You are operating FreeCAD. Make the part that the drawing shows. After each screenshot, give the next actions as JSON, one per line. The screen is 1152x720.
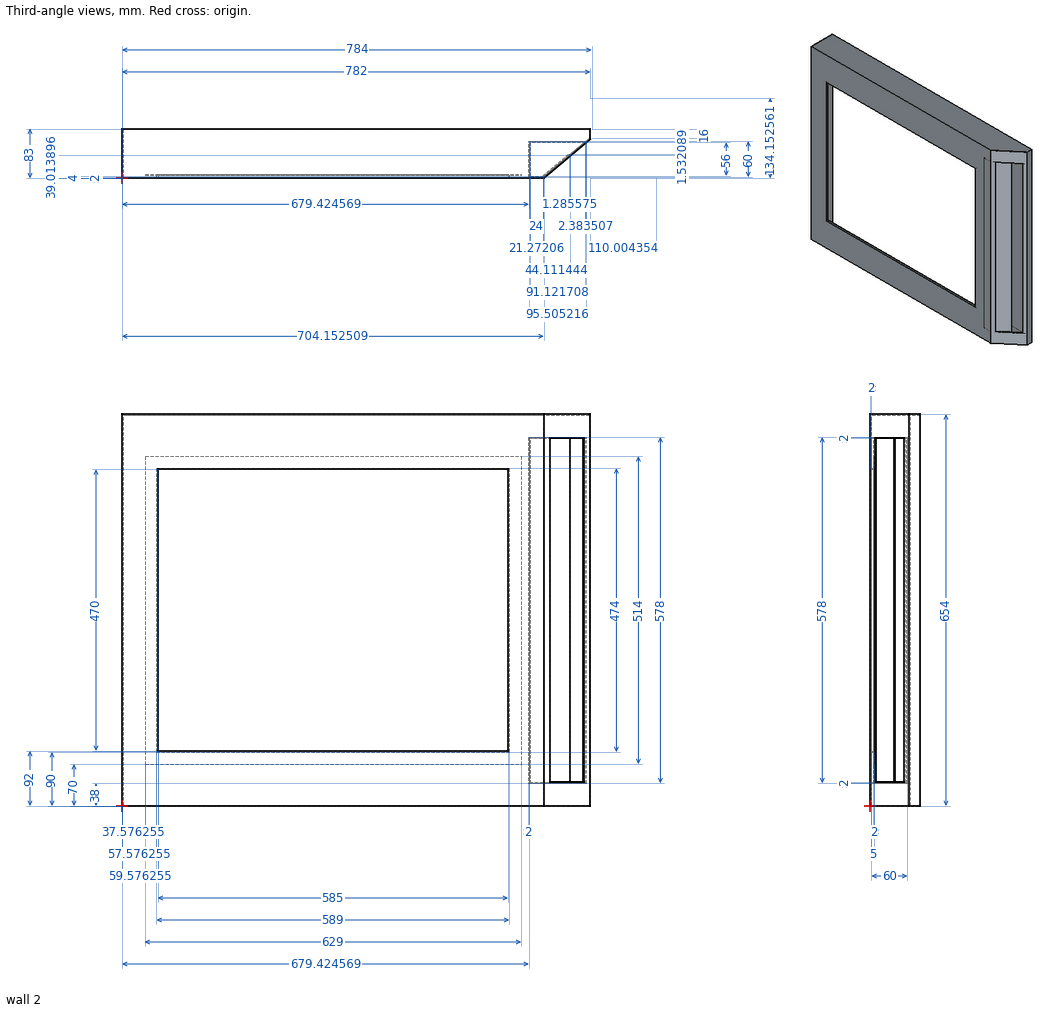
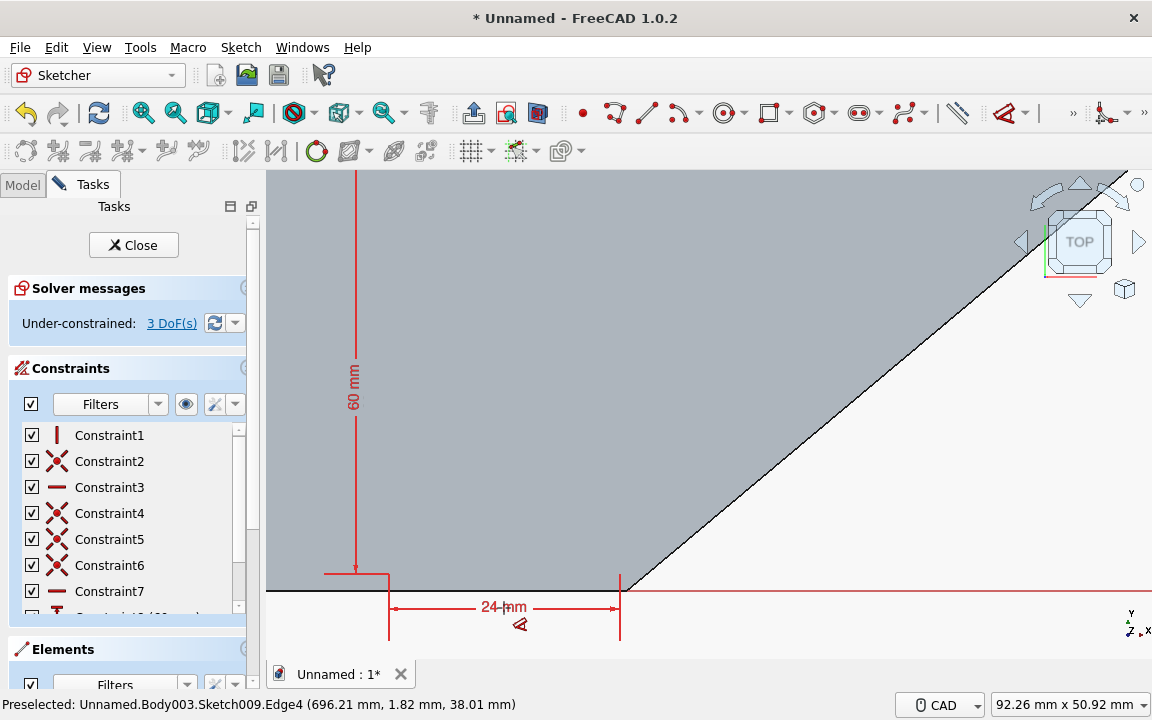
{"action": "scroll", "coordinate": [389, 574], "scroll_direction": "up", "scroll_amount": 4}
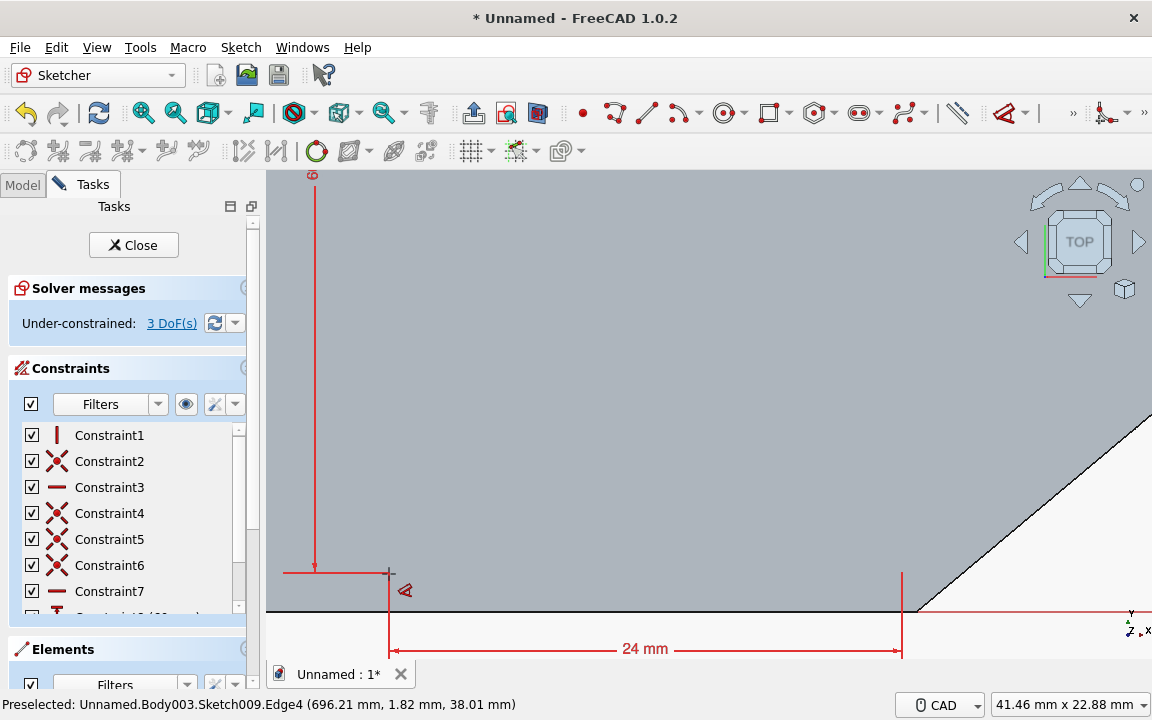
{"action": "left_click", "coordinate": [389, 573]}
{"action": "left_click", "coordinate": [423, 592]}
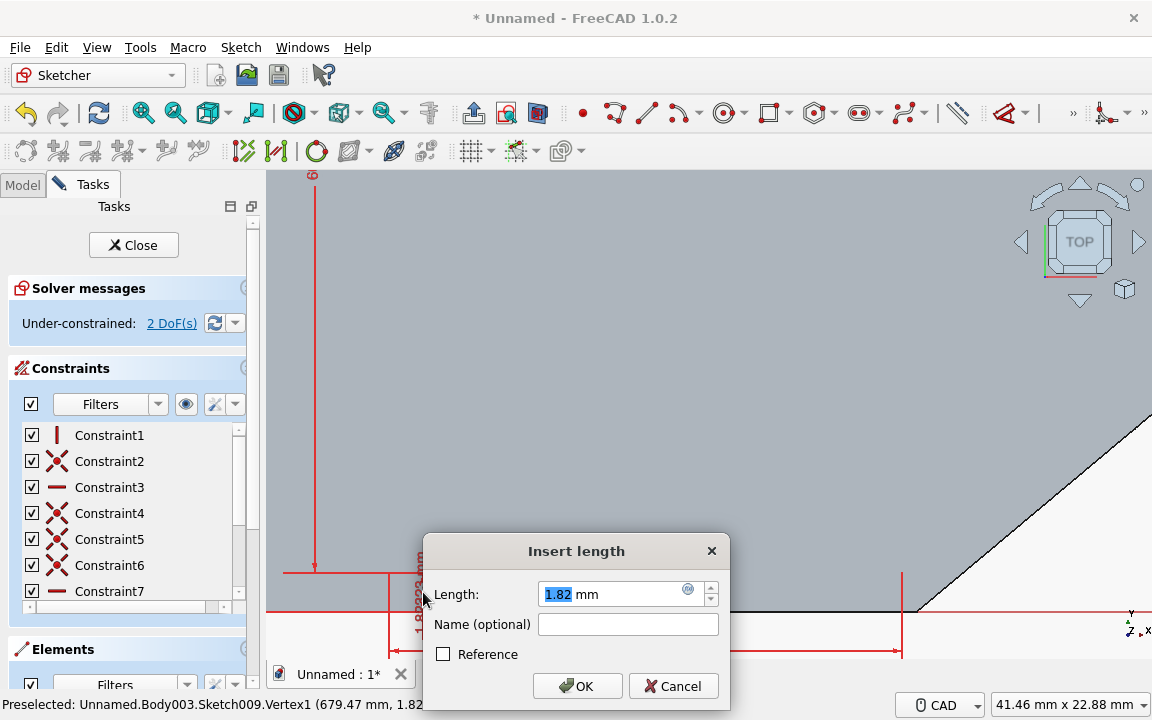
{"action": "type", "text": "2"}
{"action": "key", "text": "Return"}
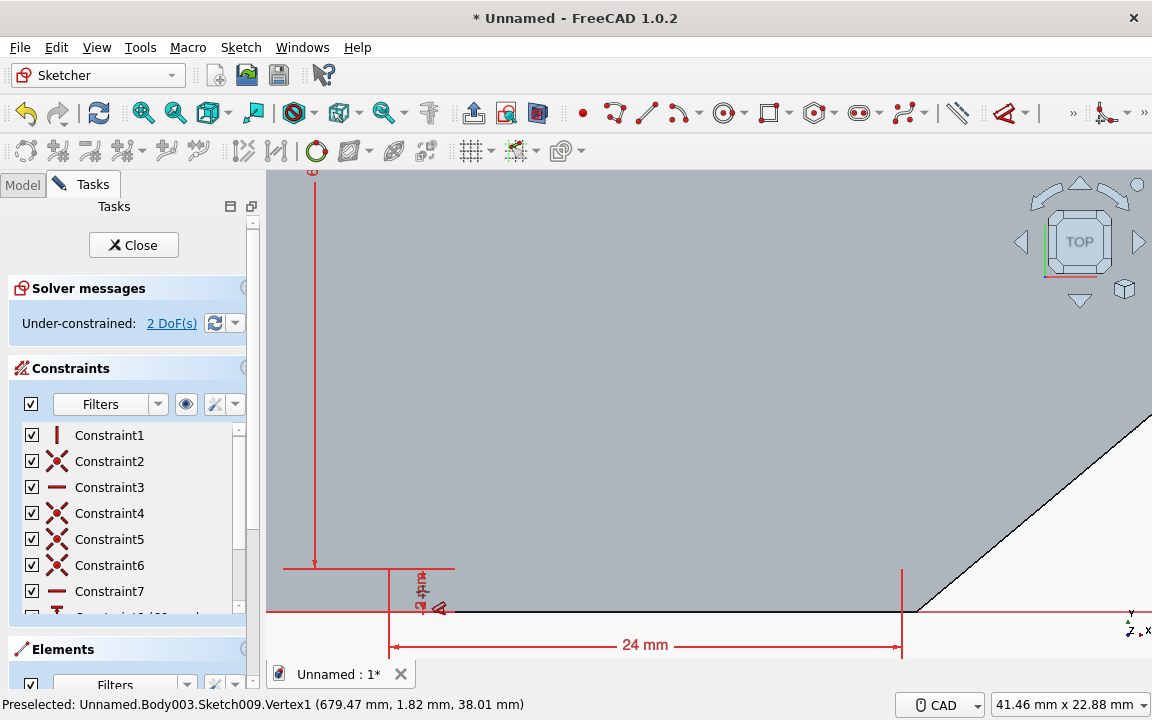
{"action": "scroll", "coordinate": [389, 574], "scroll_direction": "down", "scroll_amount": 7}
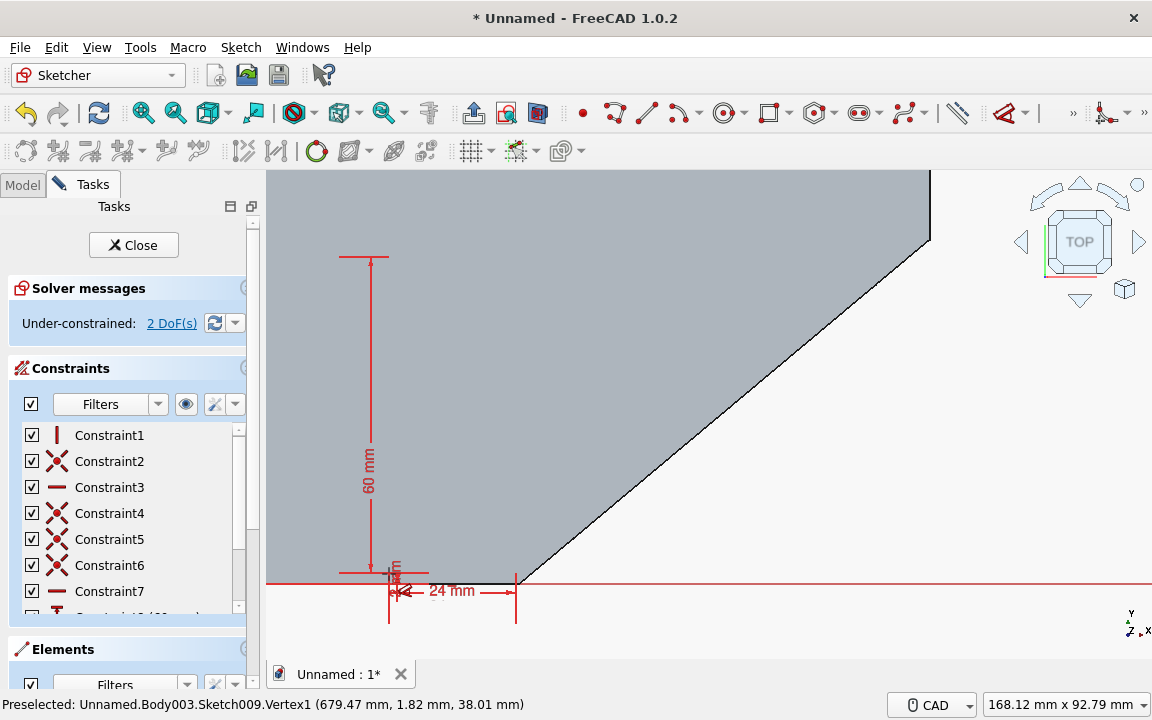
{"action": "left_click", "coordinate": [540, 257]}
{"action": "left_click", "coordinate": [641, 223]}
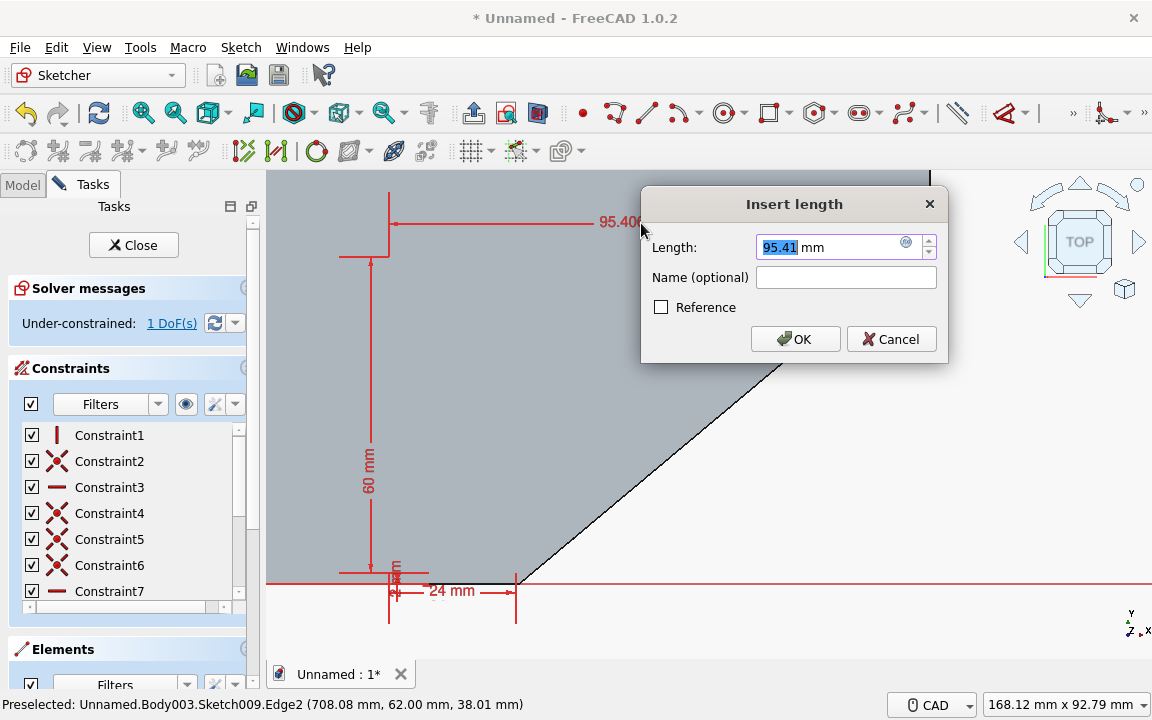
{"action": "type", "text": "95.505216"}
{"action": "key", "text": "Return"}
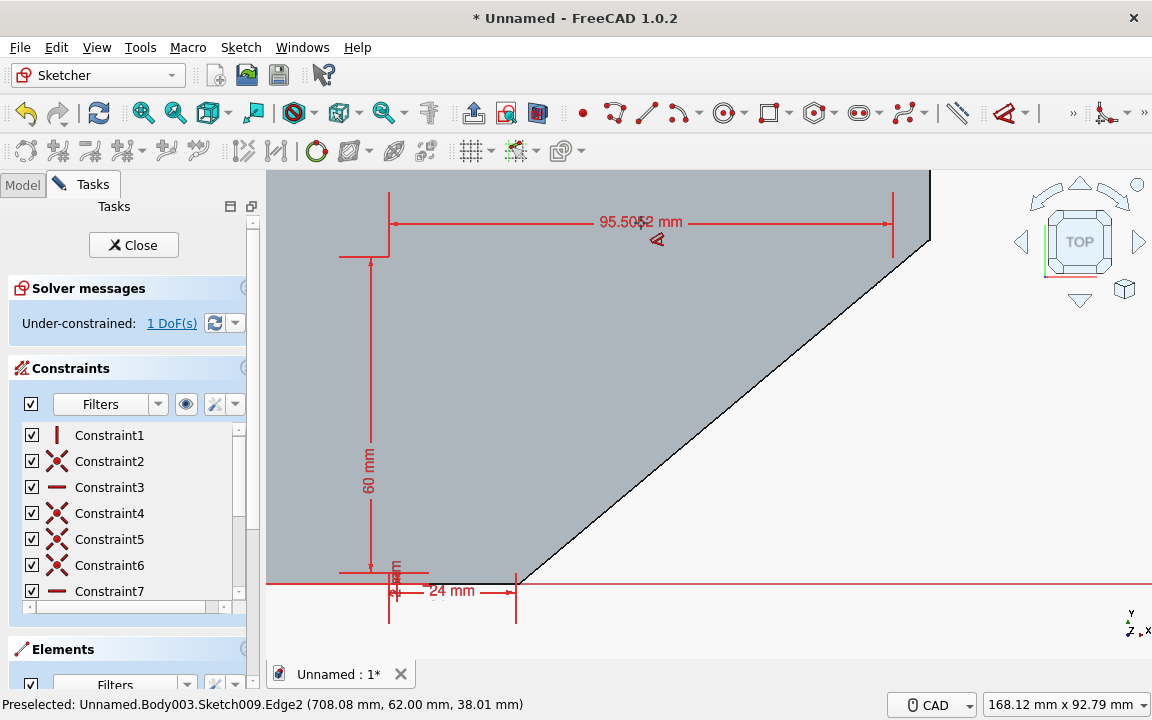
{"action": "left_click", "coordinate": [389, 573]}
{"action": "left_click", "coordinate": [342, 618]}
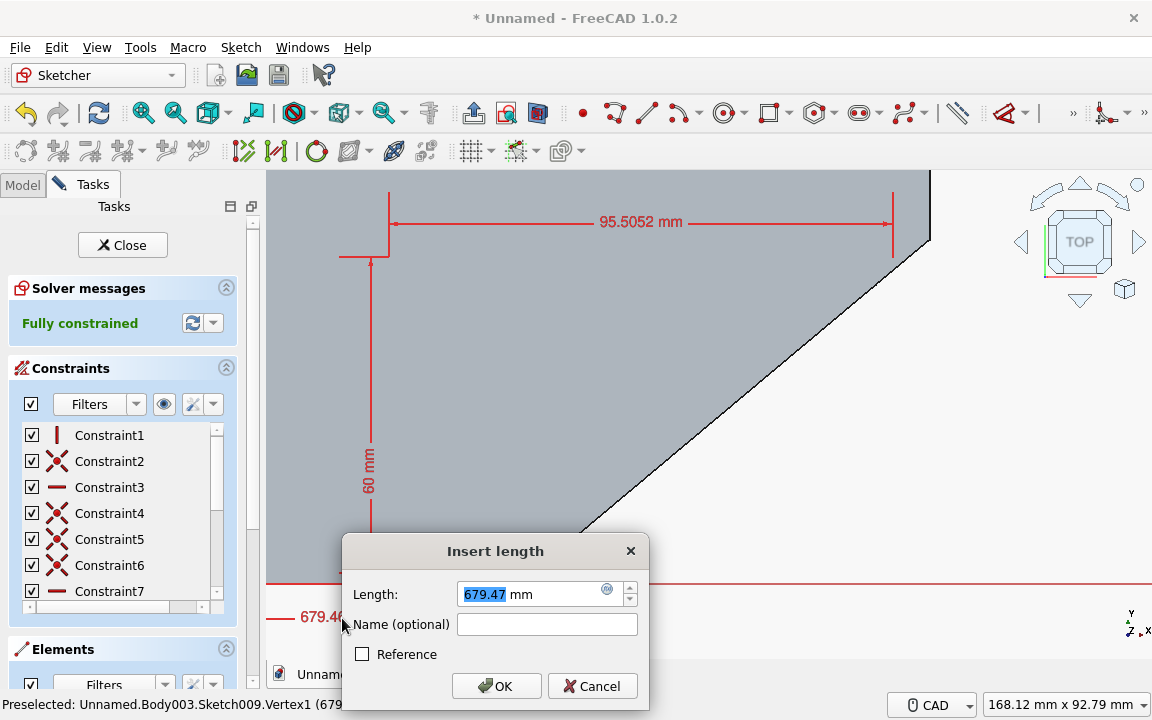
{"action": "type", "text": "679.424569"}
{"action": "key", "text": "Return"}
{"action": "key", "text": "Escape"}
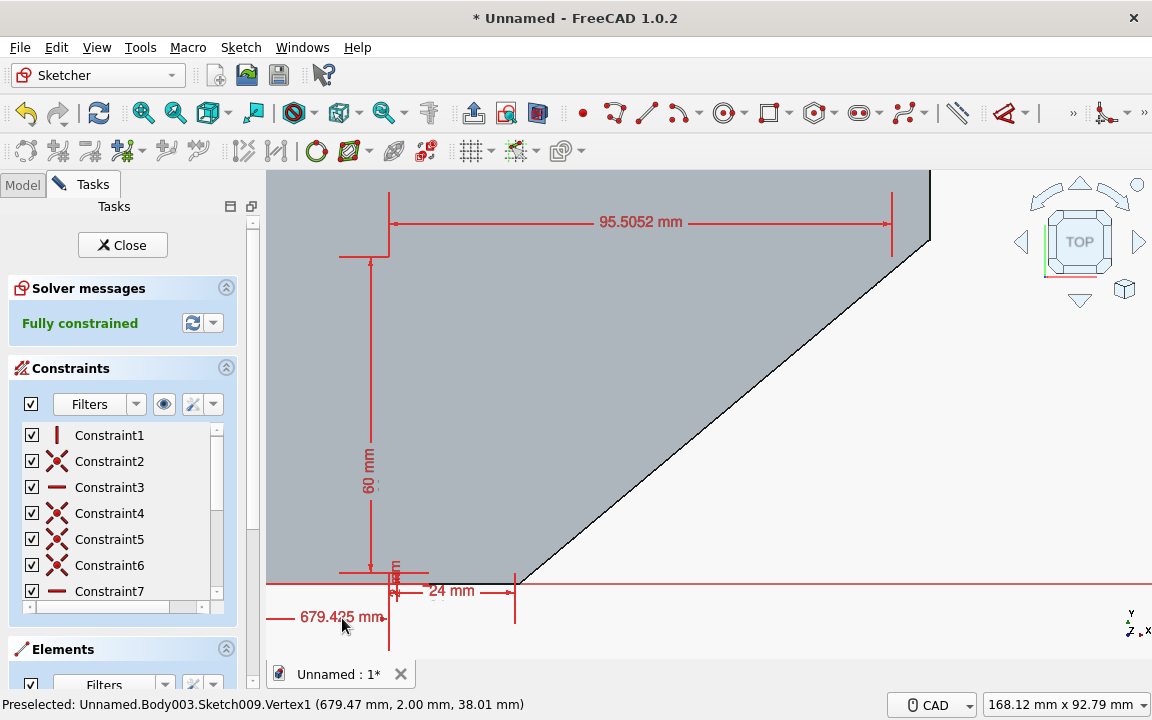
{"action": "left_click", "coordinate": [123, 245]}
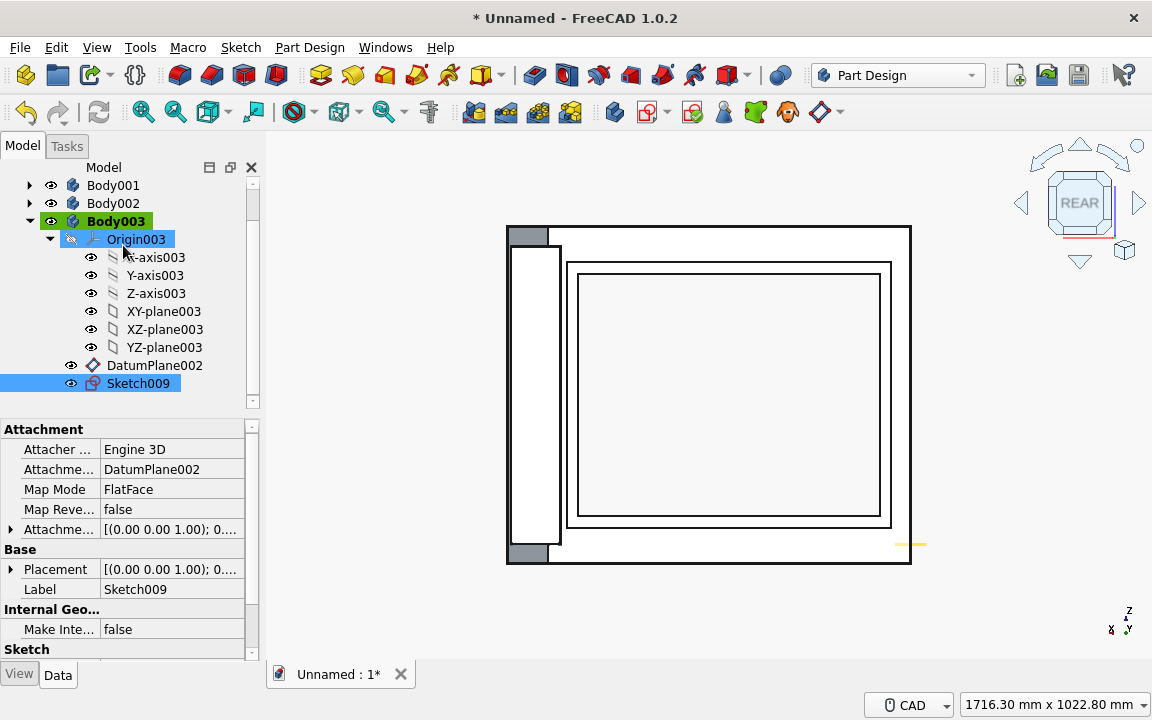
{"action": "left_click", "coordinate": [322, 76]}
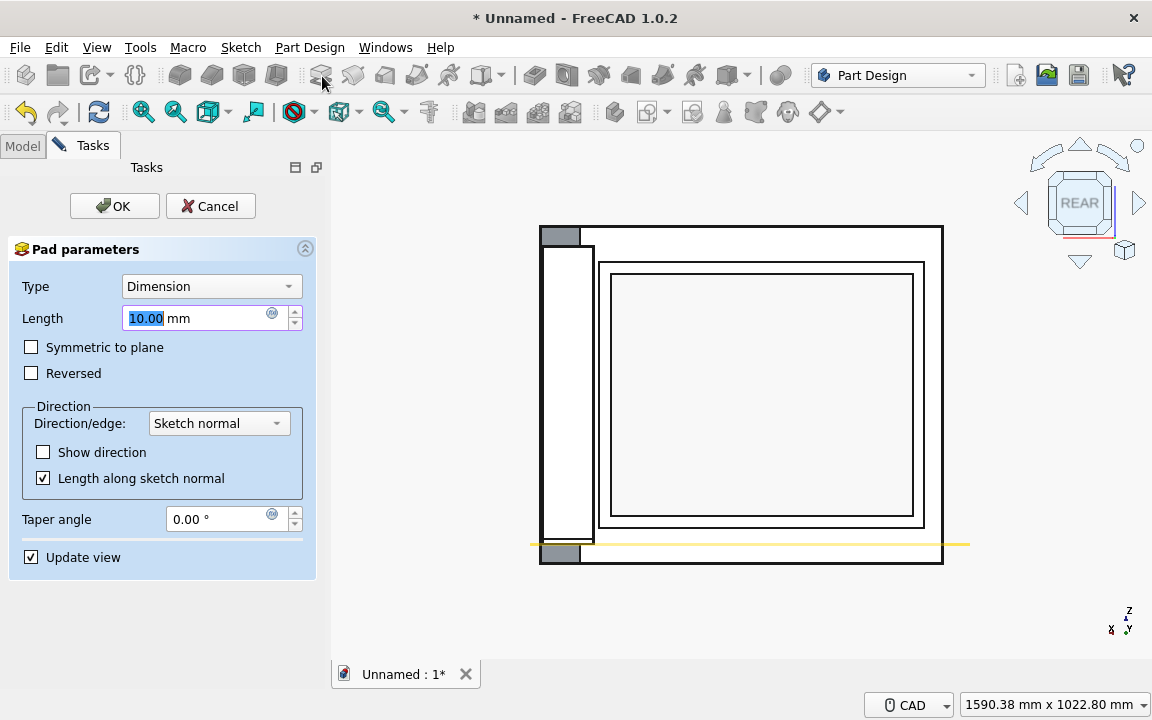
{"action": "type", "text": "2"}
{"action": "key", "text": "Tab"}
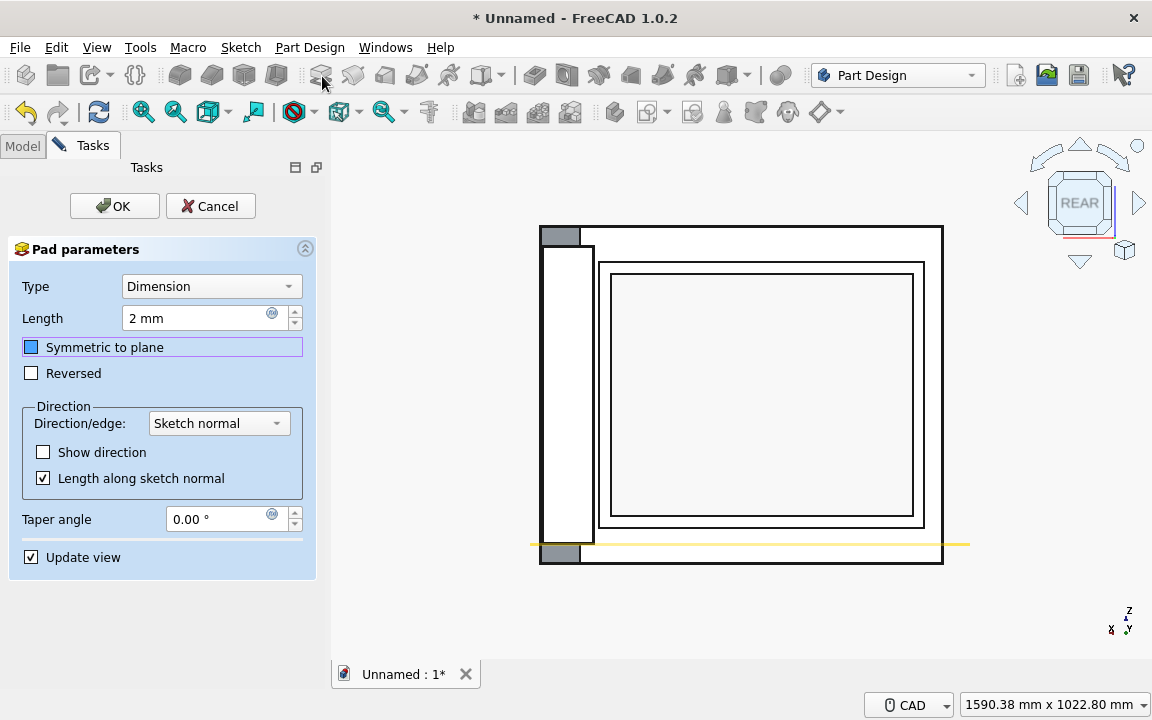
{"action": "left_click", "coordinate": [115, 206]}